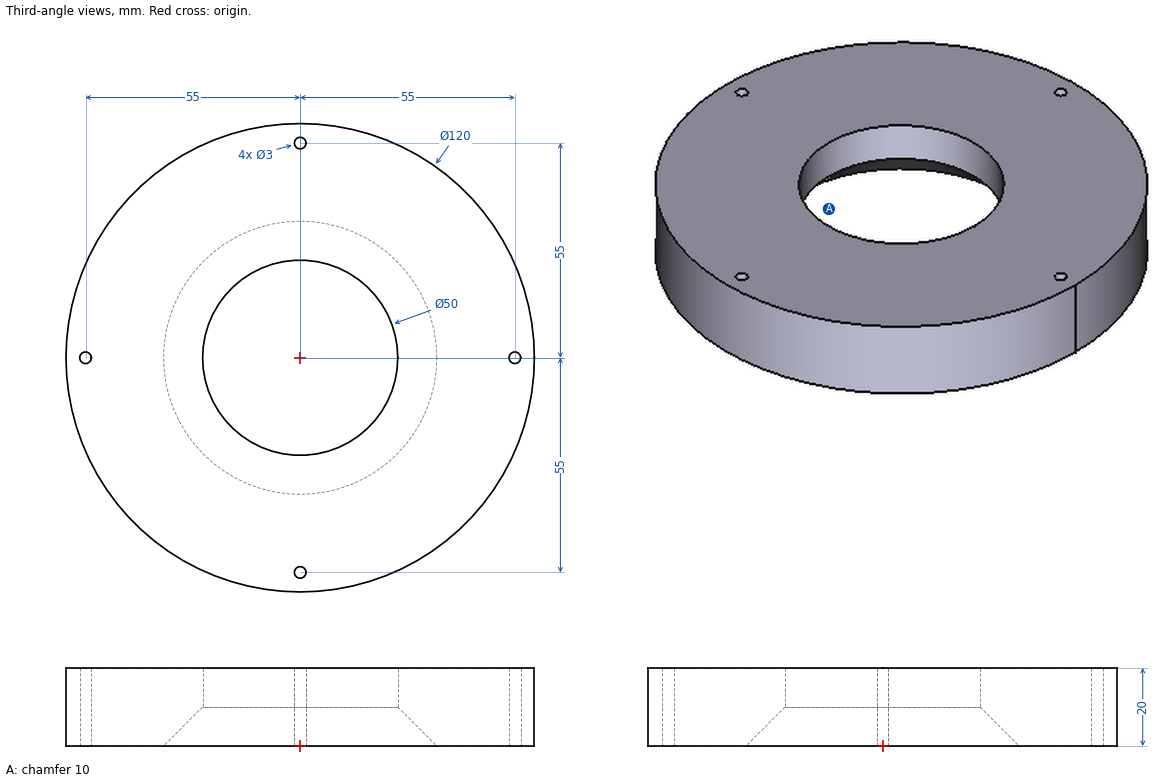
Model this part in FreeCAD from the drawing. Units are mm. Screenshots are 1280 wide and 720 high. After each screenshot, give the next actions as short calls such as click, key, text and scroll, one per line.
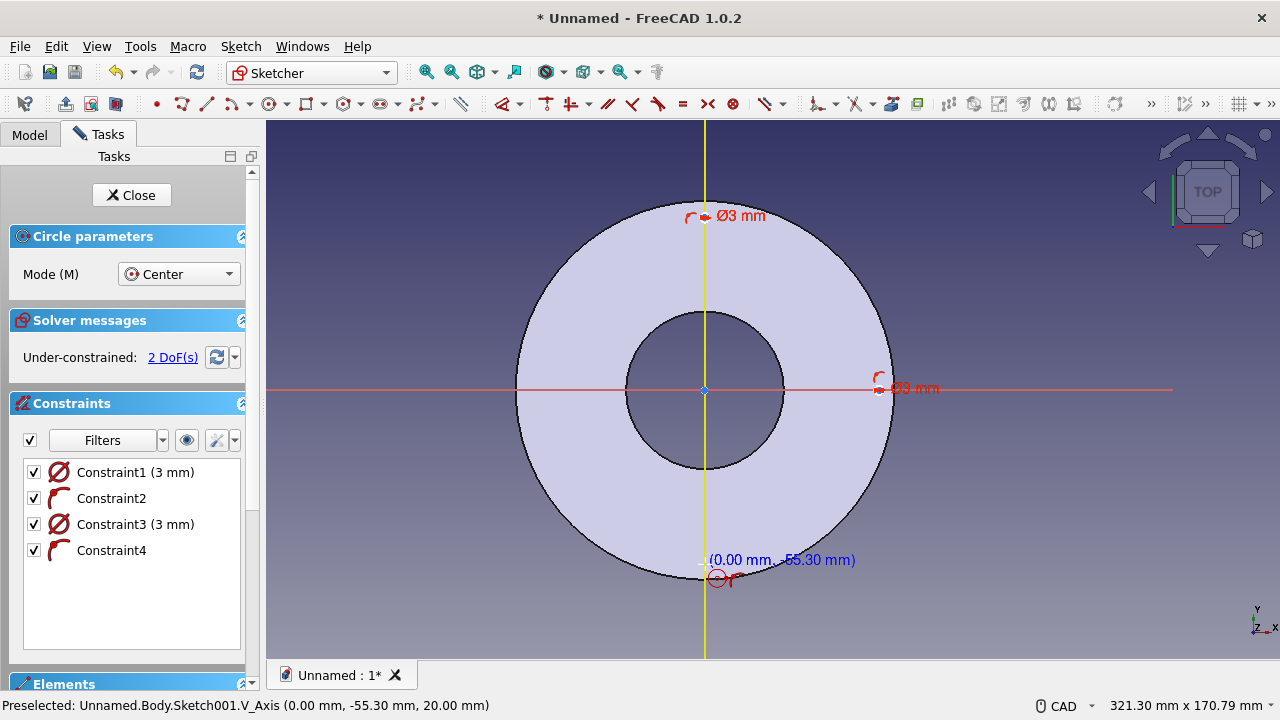
click(705, 564)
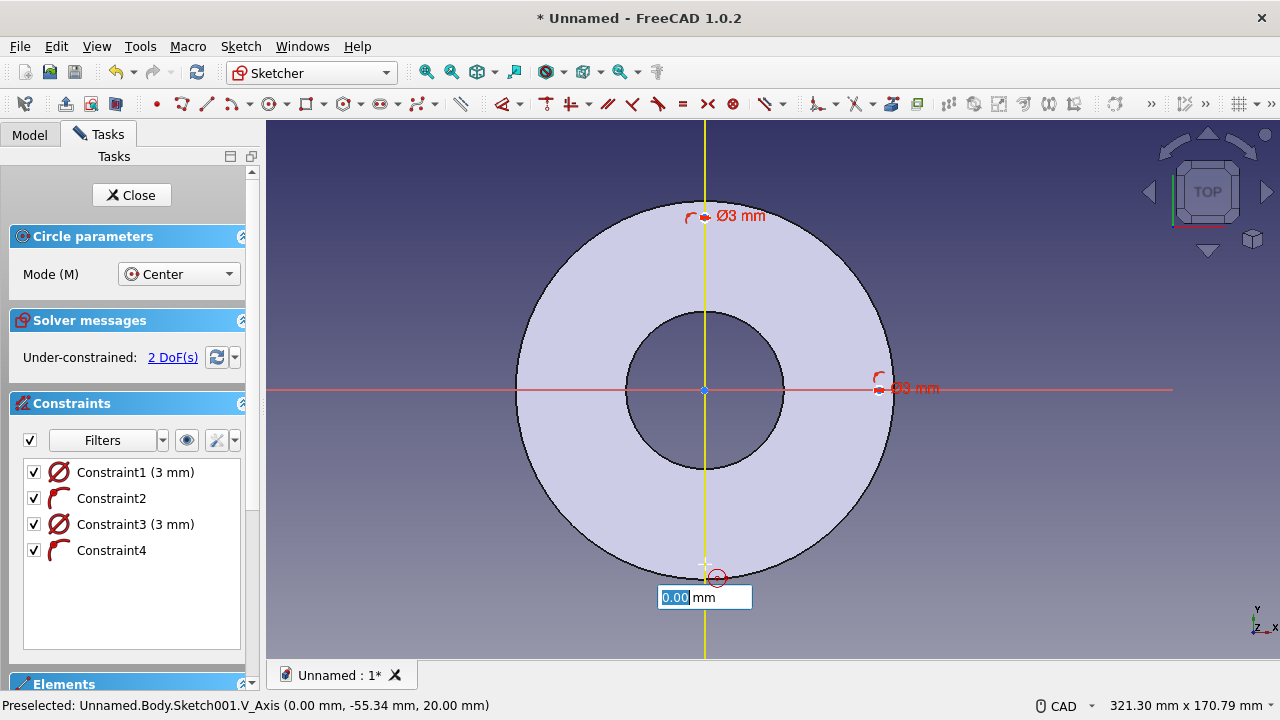
scroll(709, 562, up, 7)
move(709, 561)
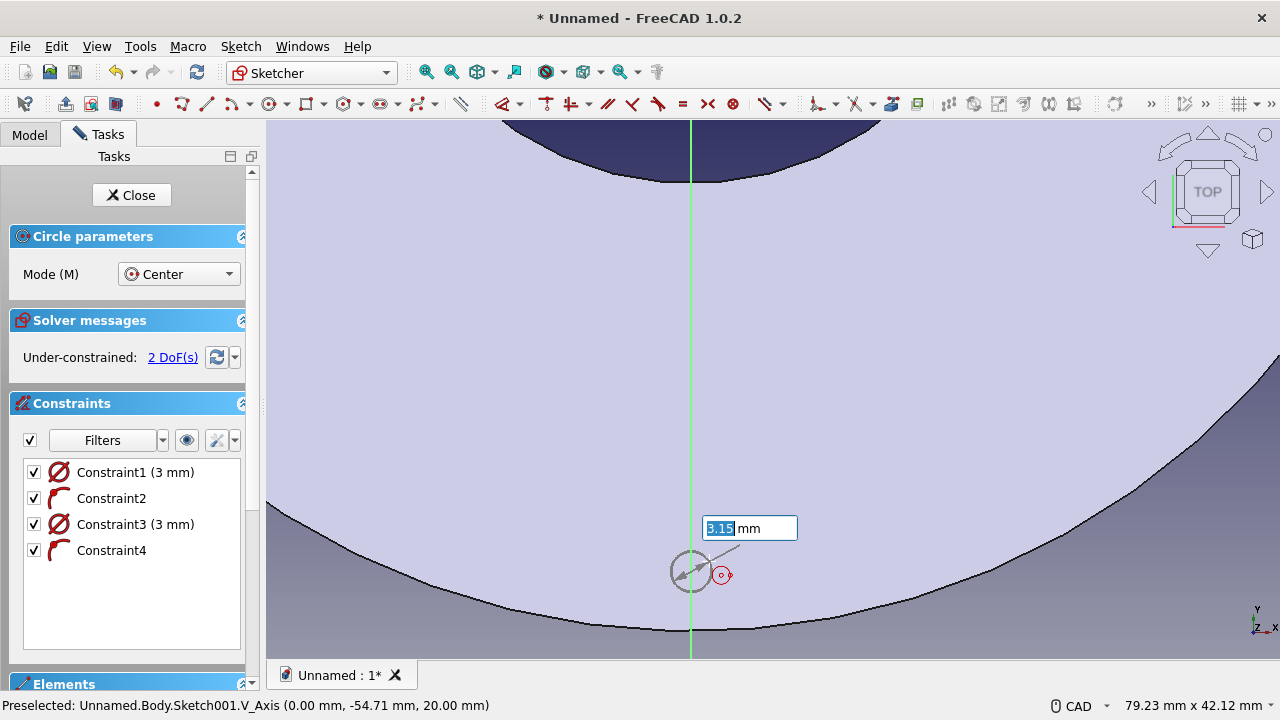
text(3)
key(Return)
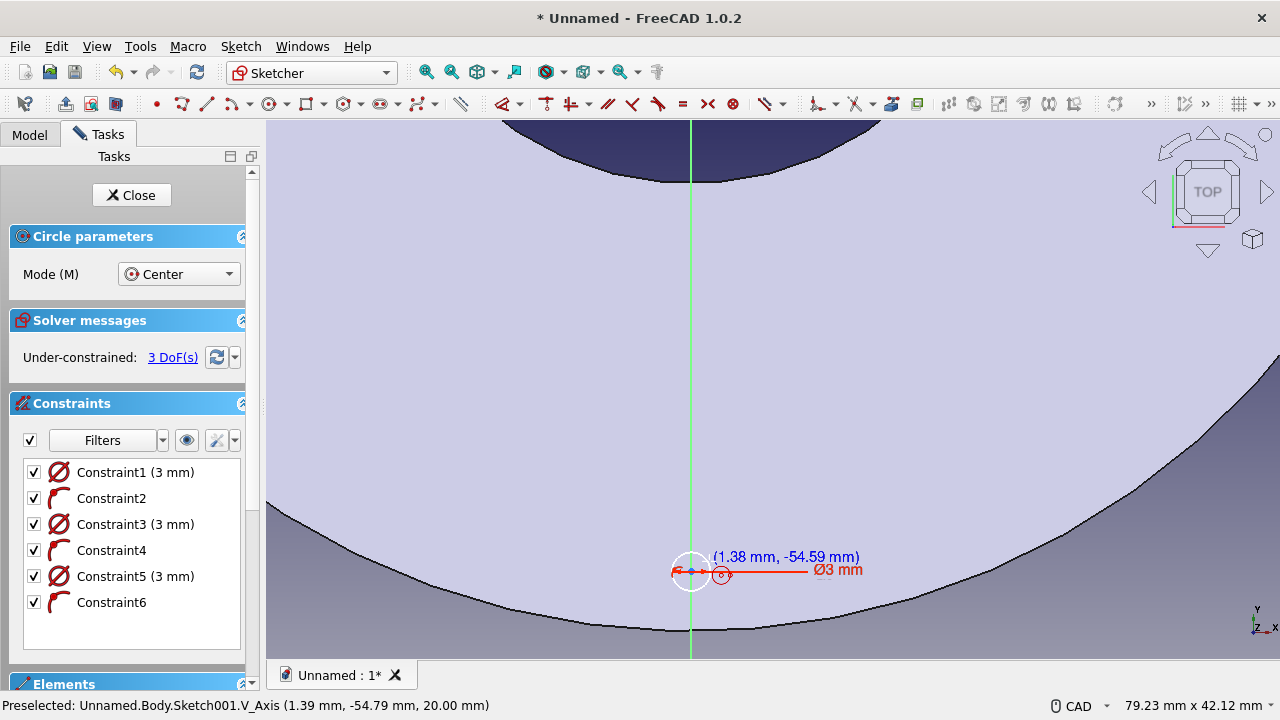
scroll(709, 562, down, 7)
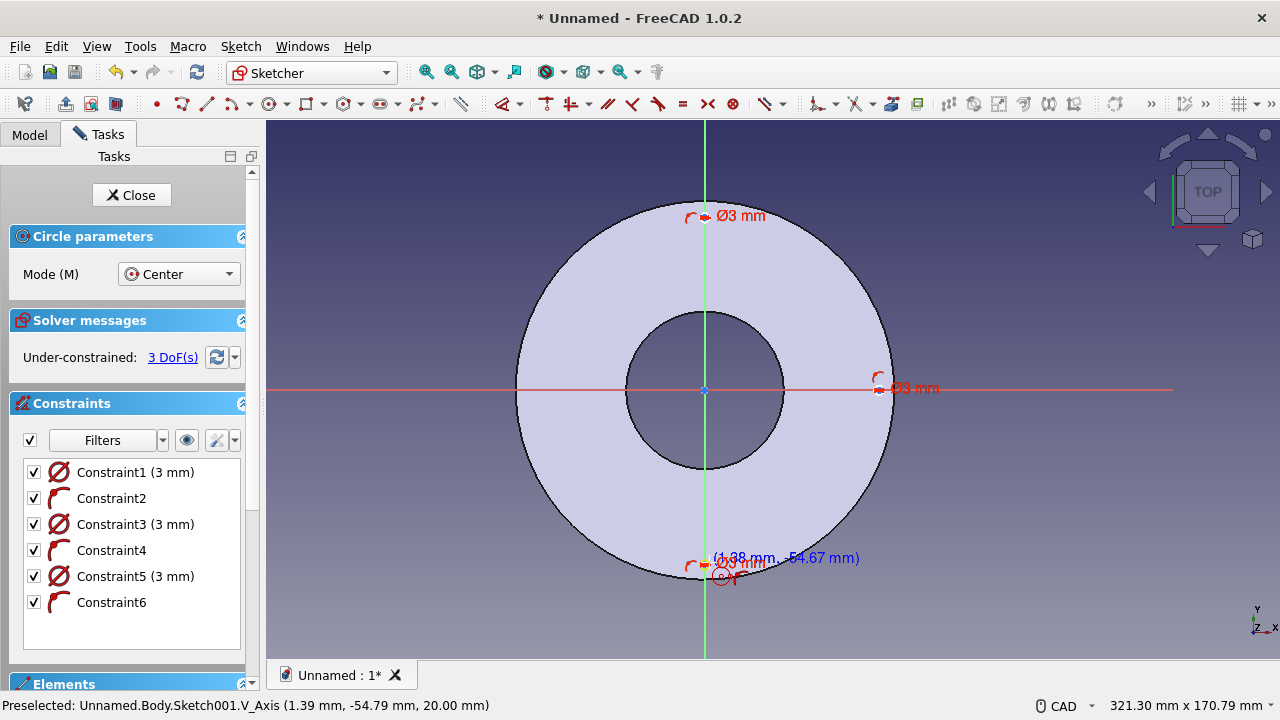
scroll(531, 390, up, 8)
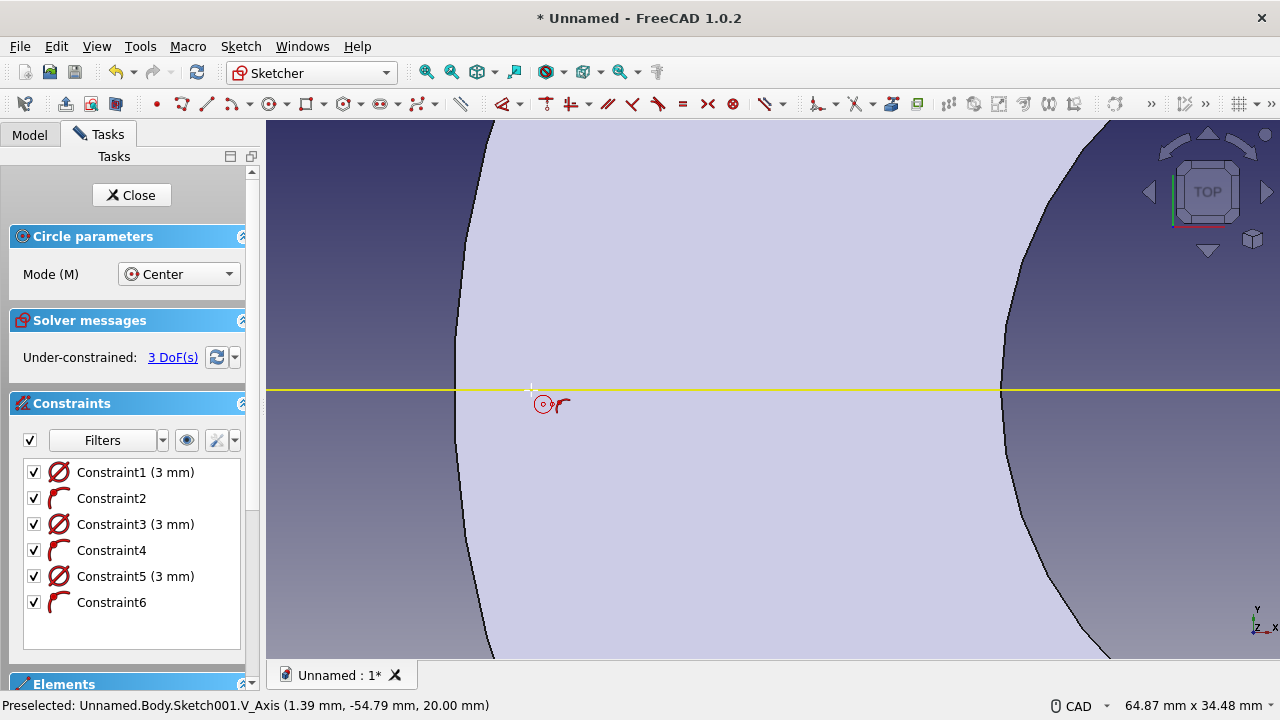
scroll(531, 389, down, 8)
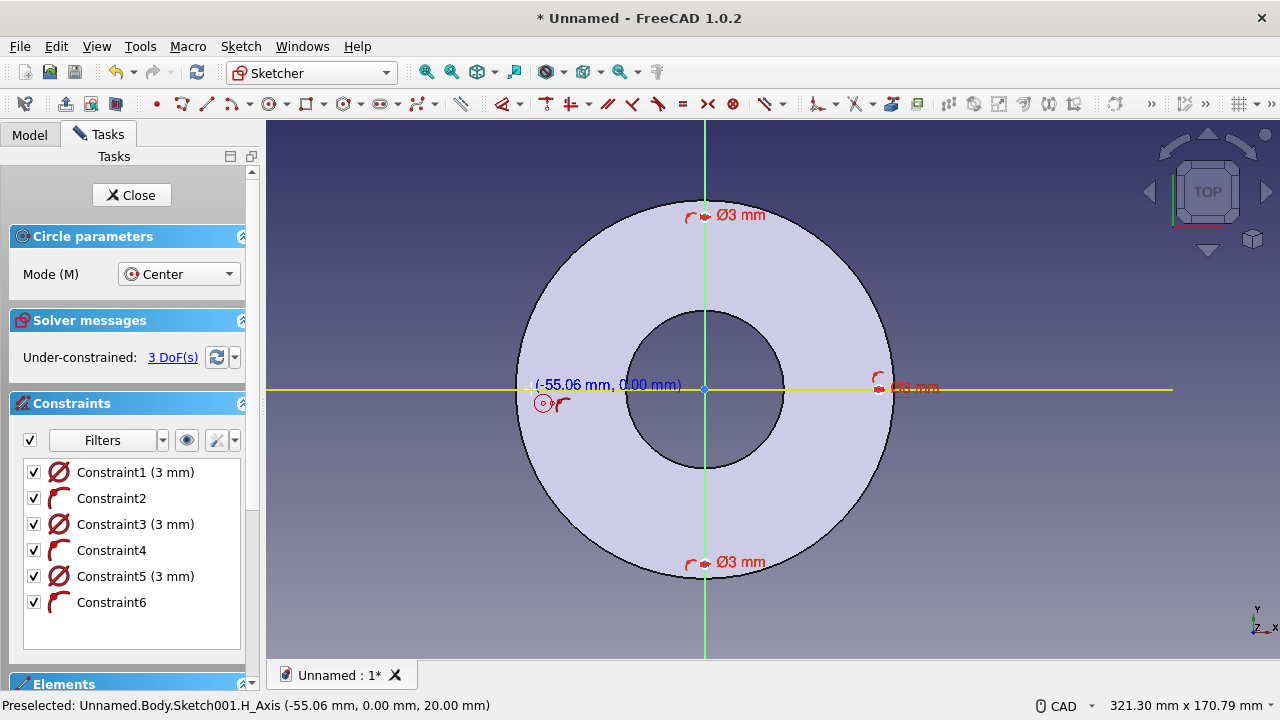
click(531, 390)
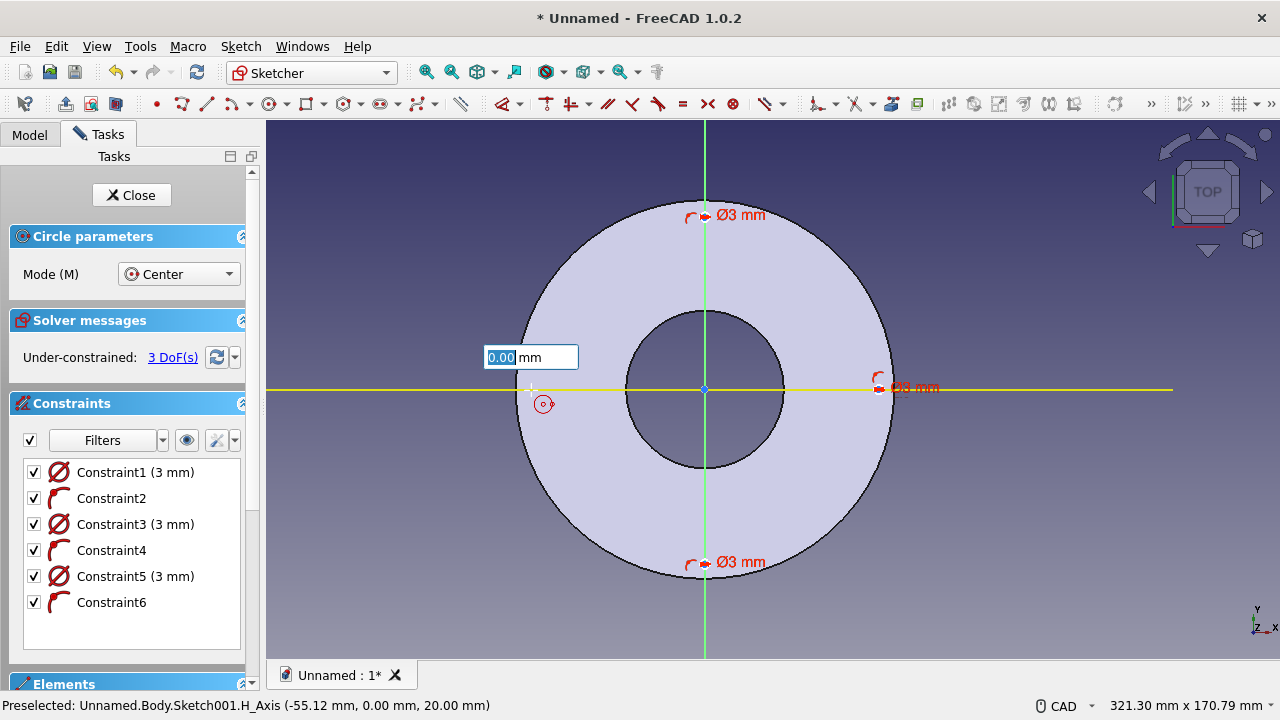
scroll(530, 394, up, 7)
move(528, 392)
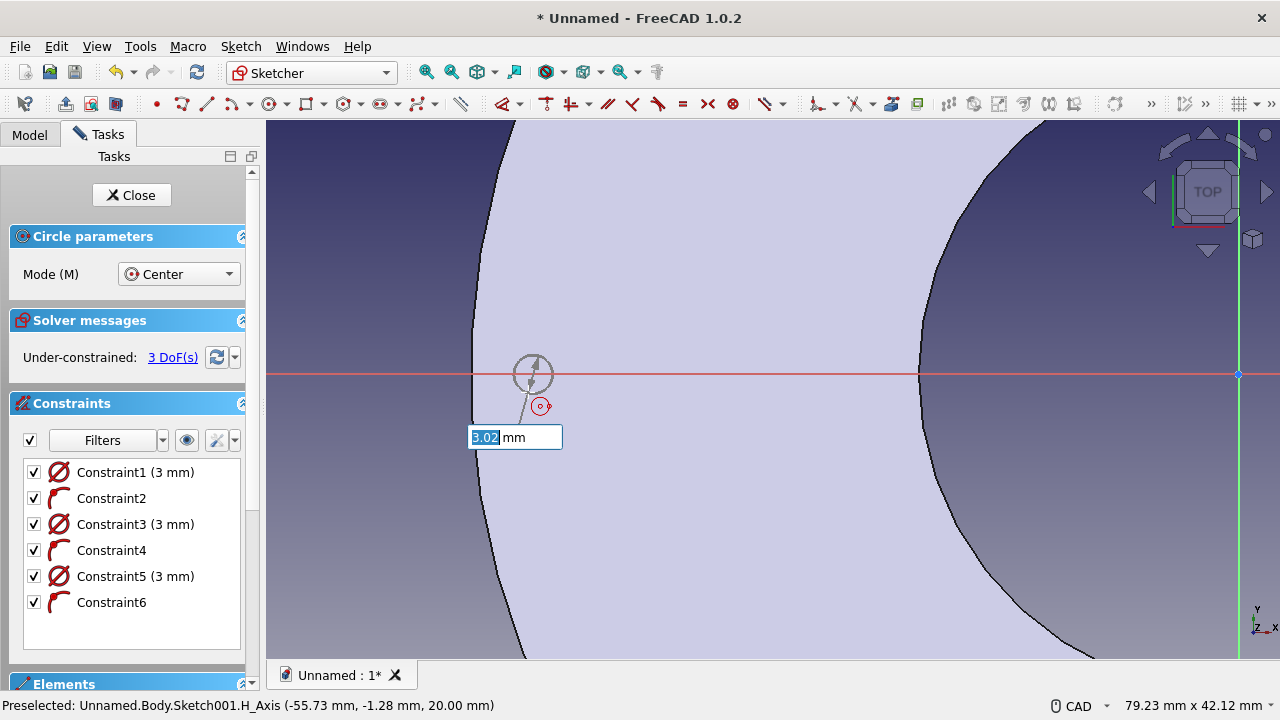
text(3)
key(Return)
key(Escape)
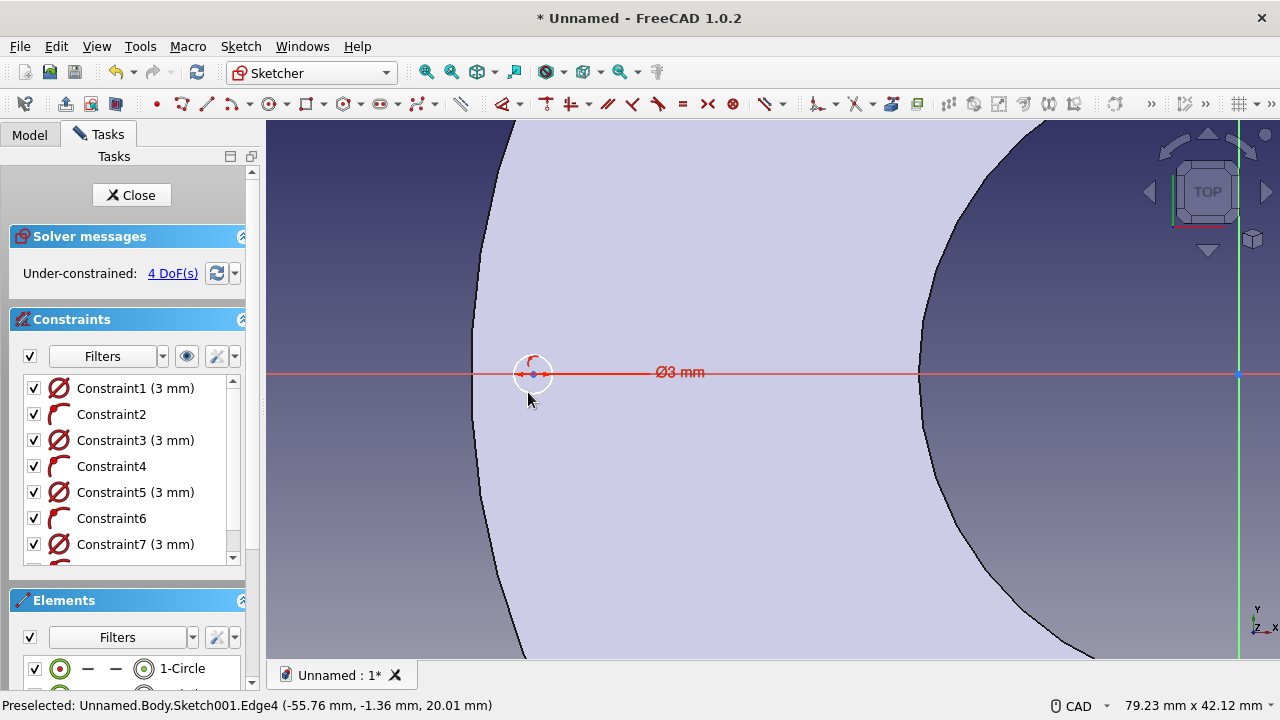
key(d)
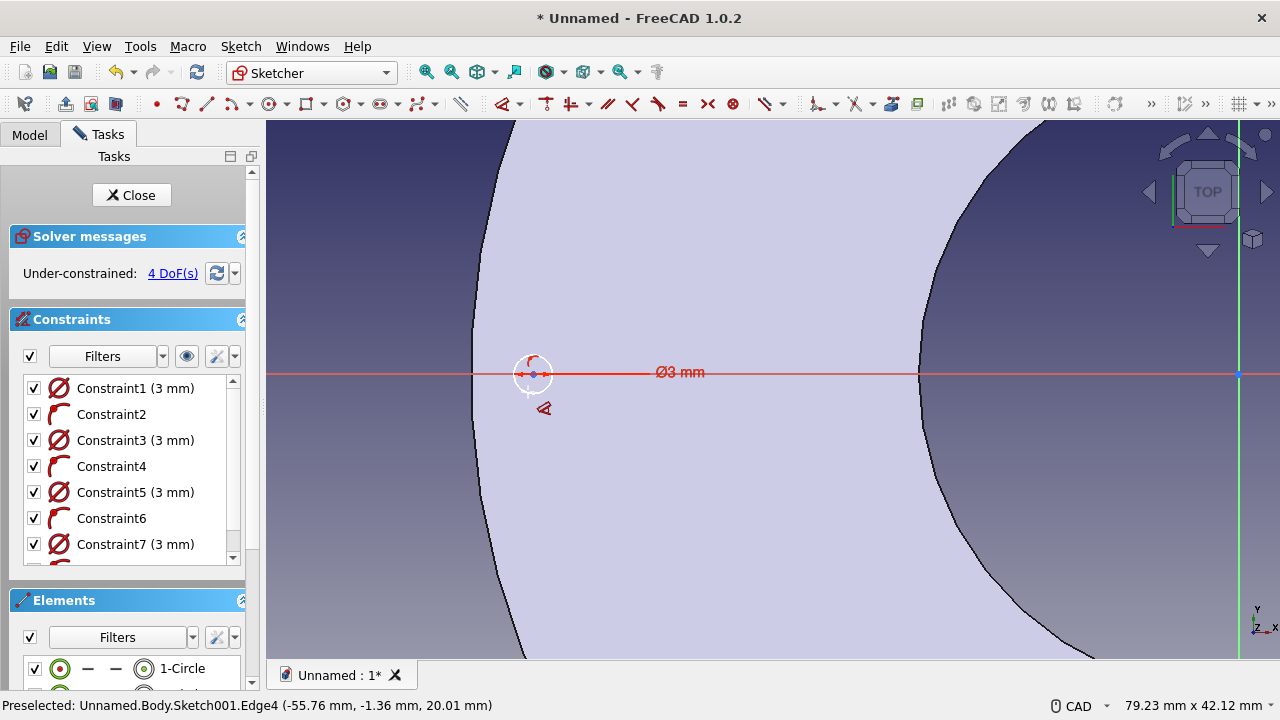
scroll(530, 394, down, 7)